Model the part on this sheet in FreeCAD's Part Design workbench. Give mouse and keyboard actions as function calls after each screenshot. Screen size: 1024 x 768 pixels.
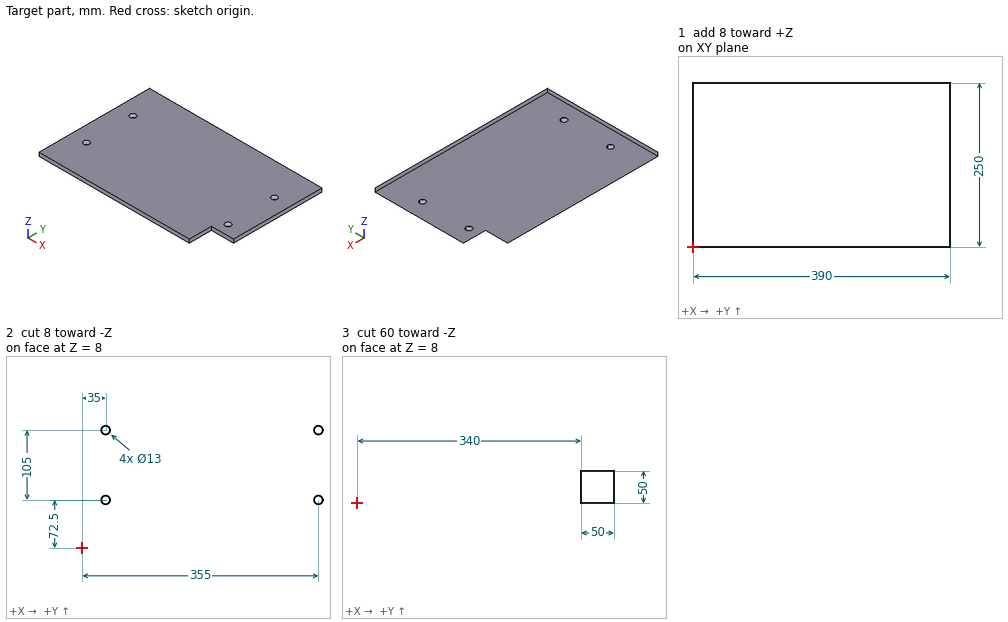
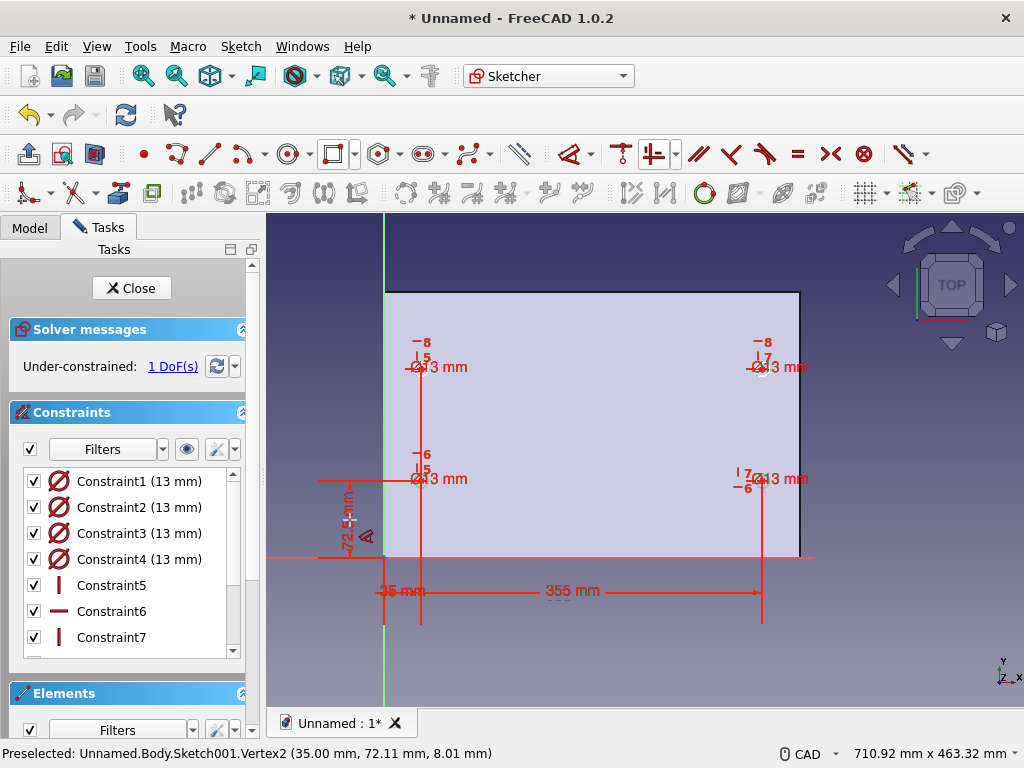
click(421, 369)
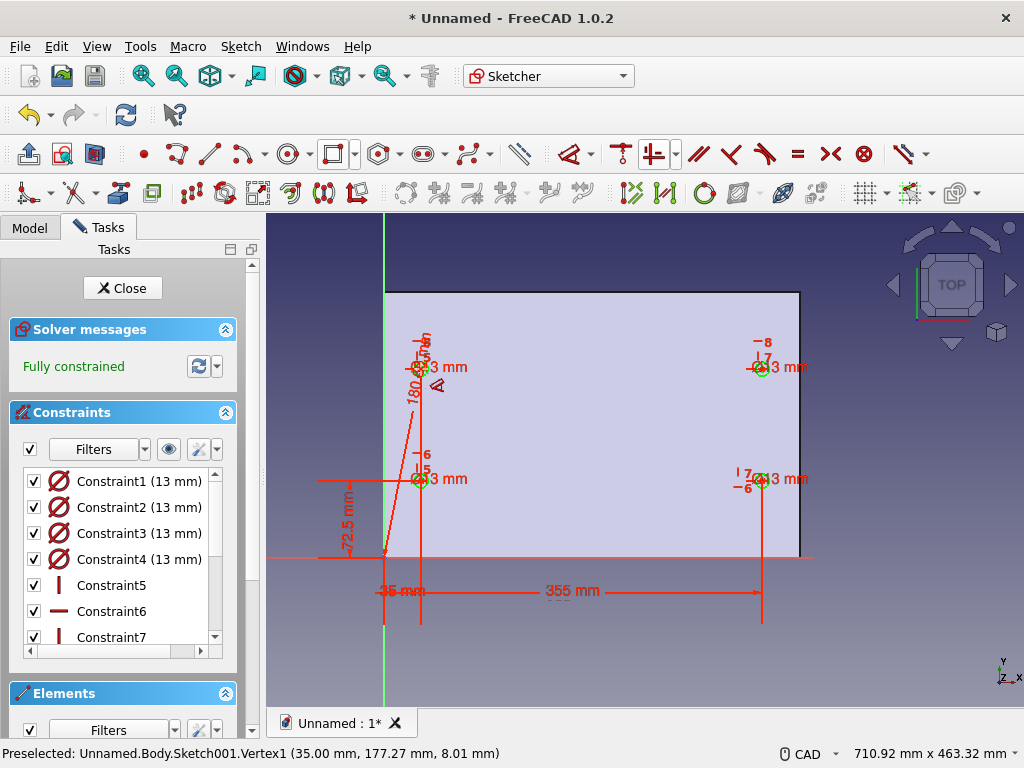
click(421, 481)
click(455, 425)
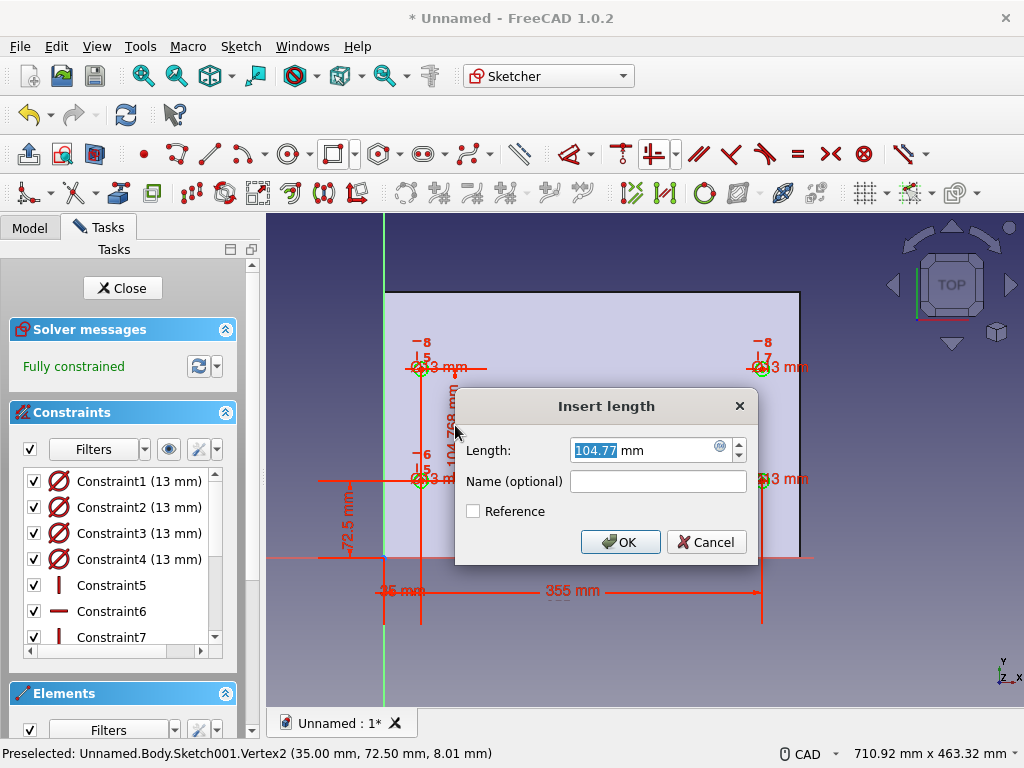
text(105)
key(Return)
key(Escape)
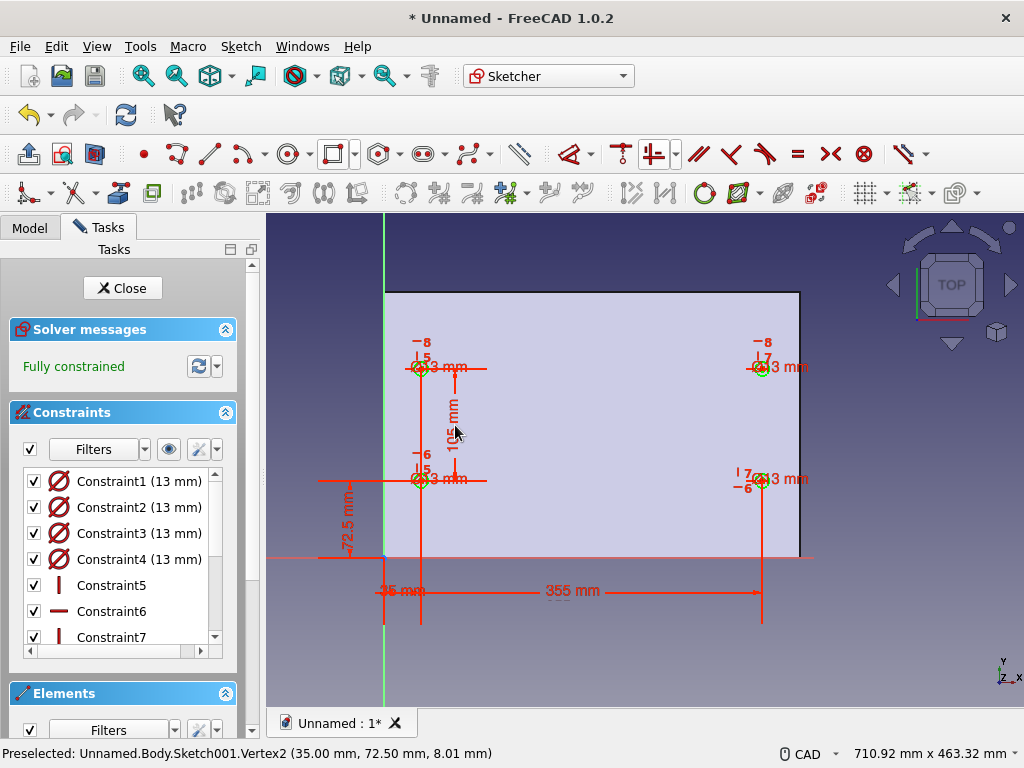
click(123, 288)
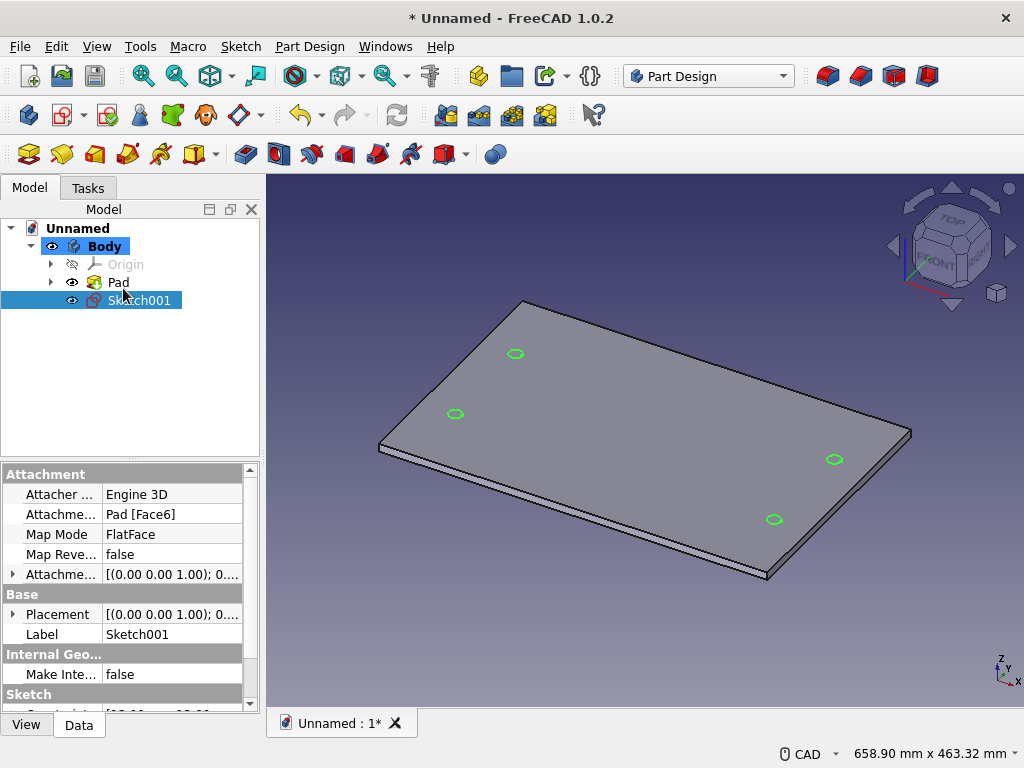
click(246, 154)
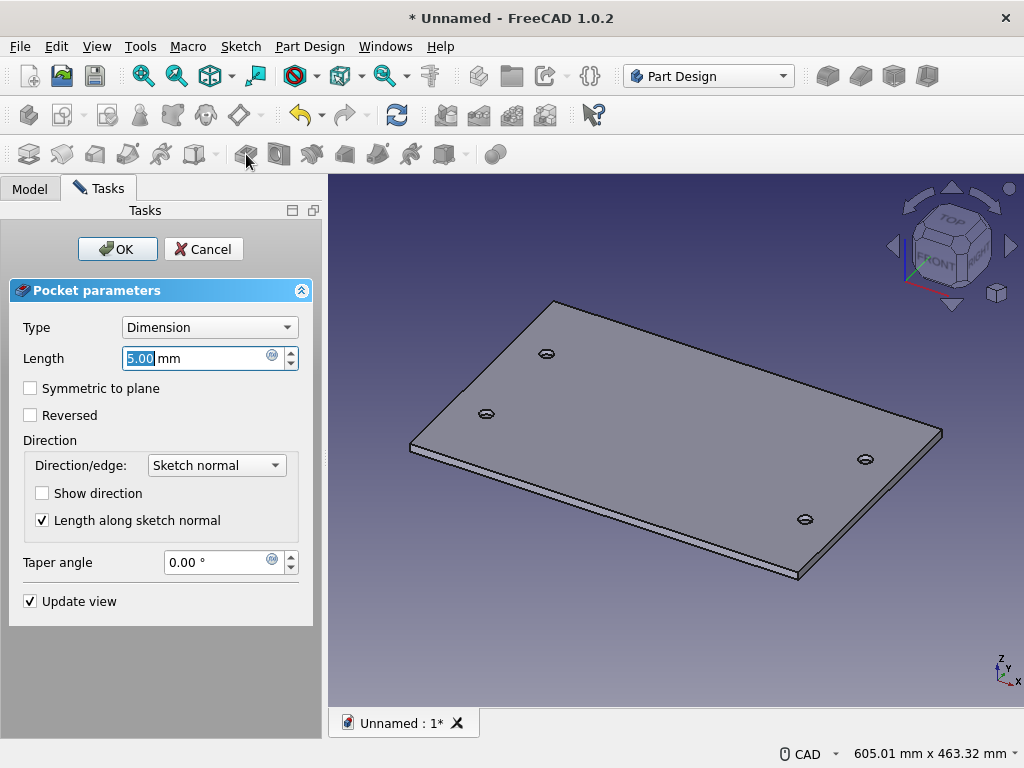
text(8)
key(Tab)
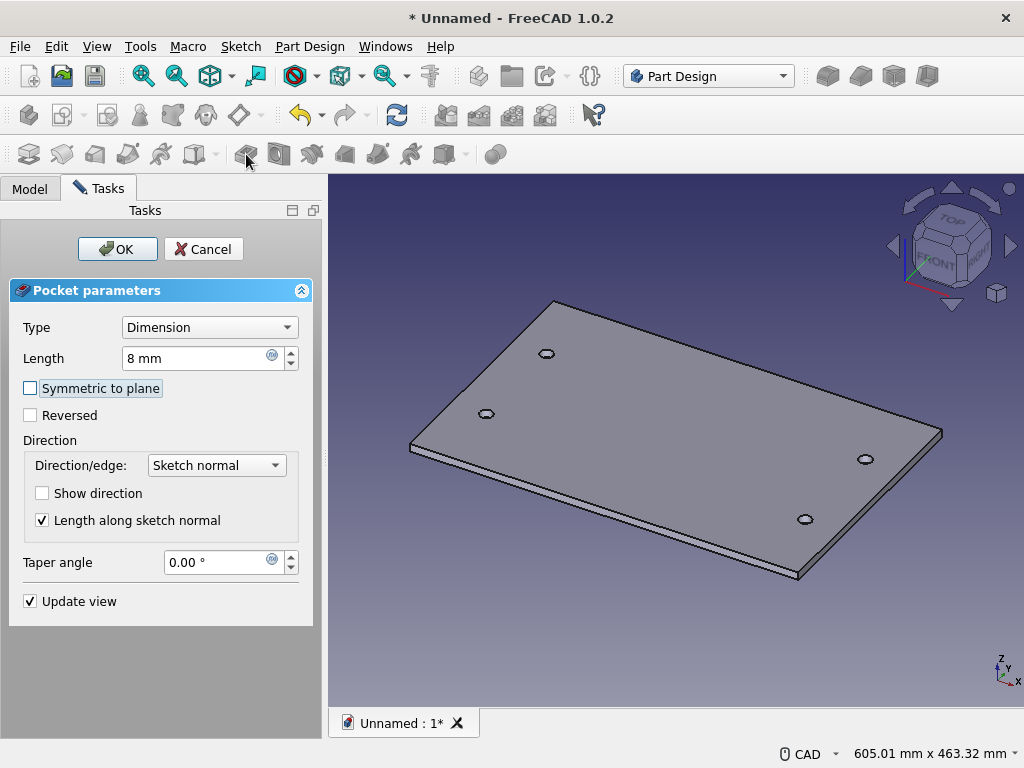
click(118, 249)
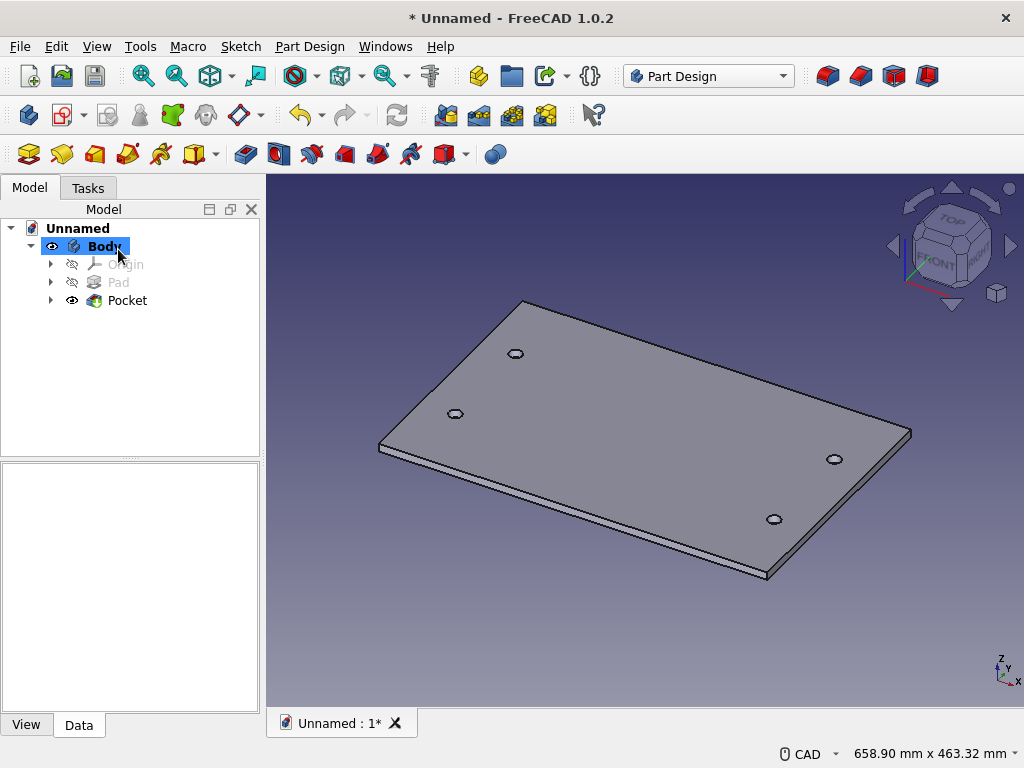
click(645, 436)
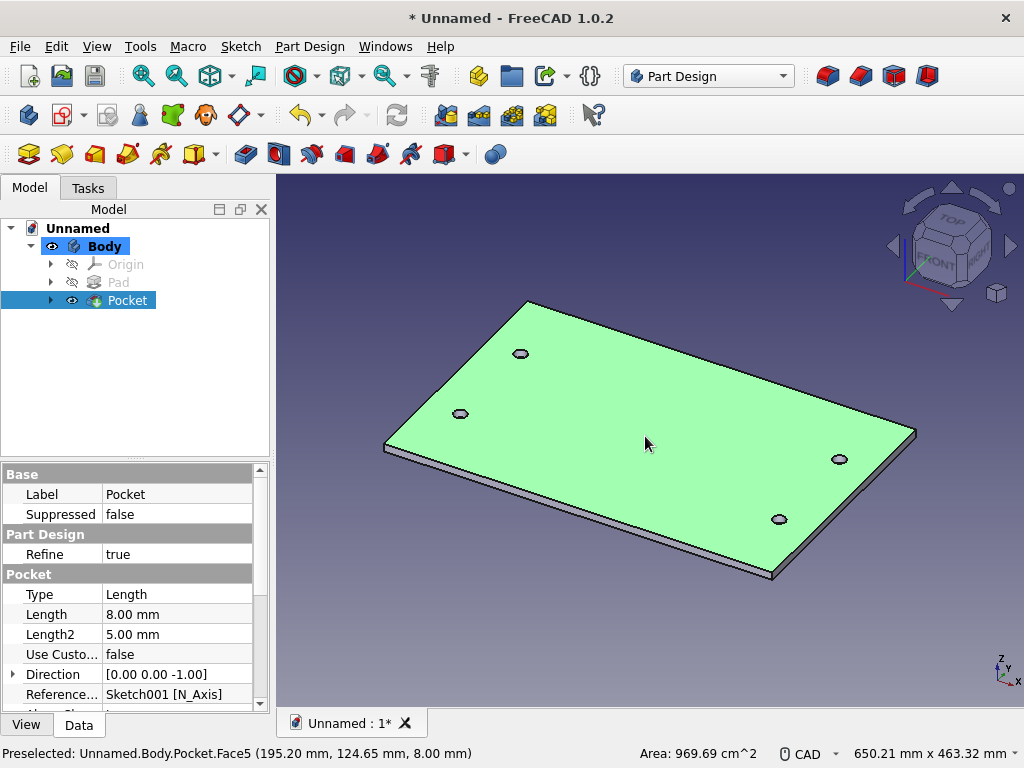
click(62, 116)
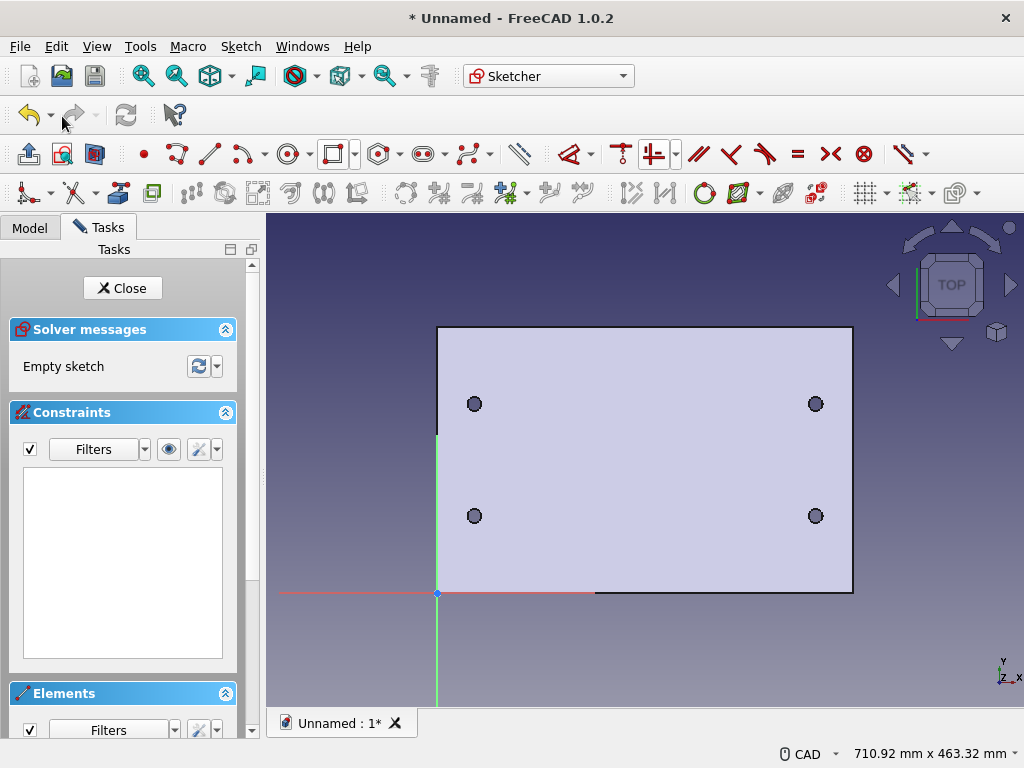
scroll(859, 588, up, 9)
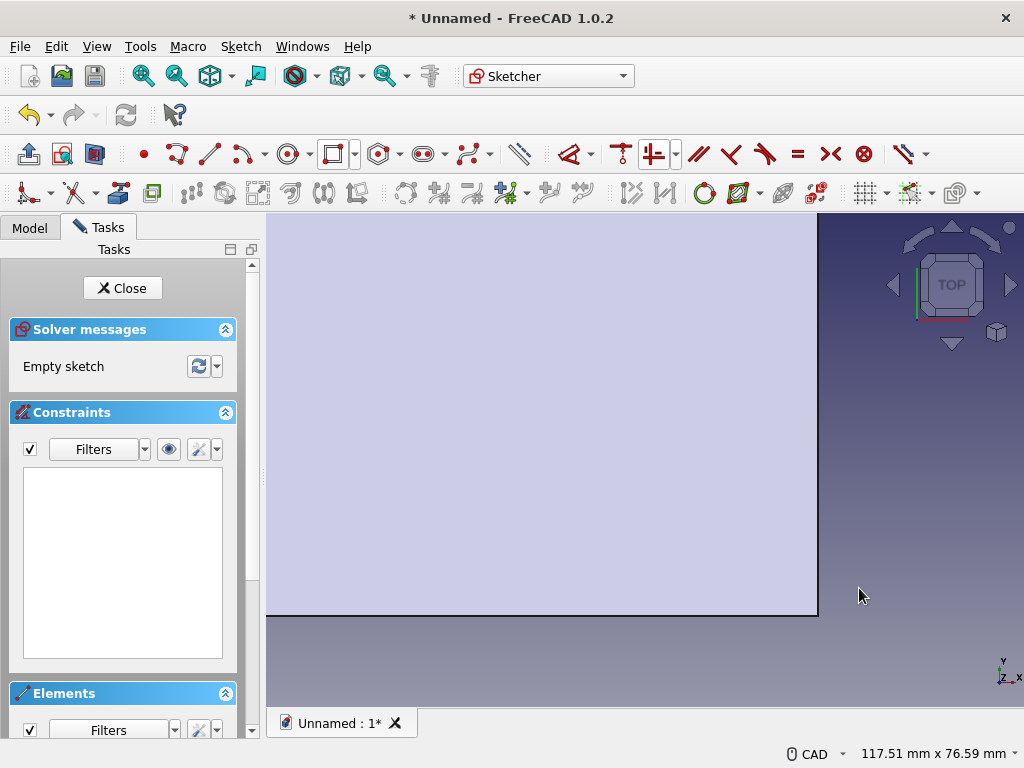
click(332, 154)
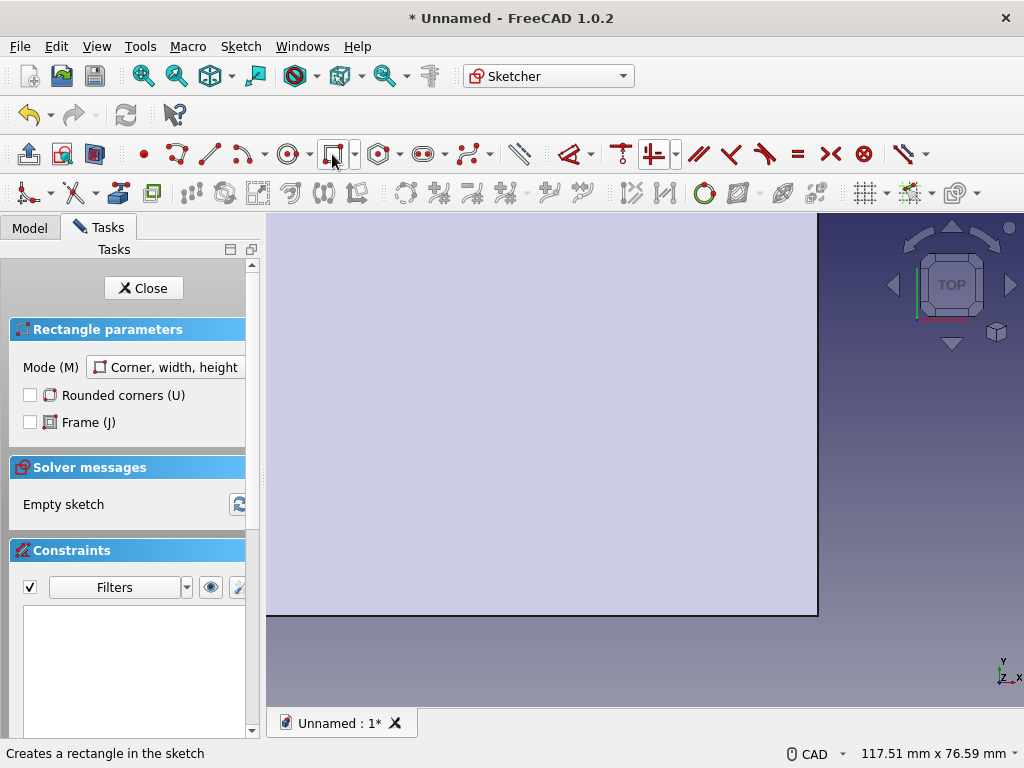
click(496, 294)
click(818, 616)
key(Escape)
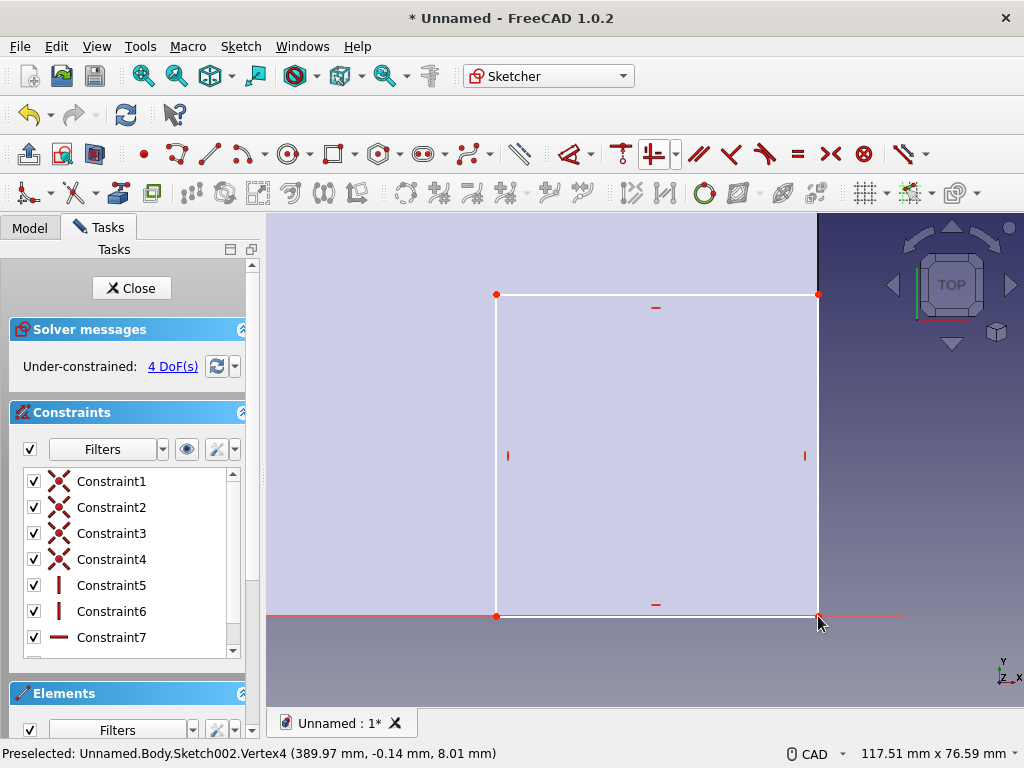
click(496, 617)